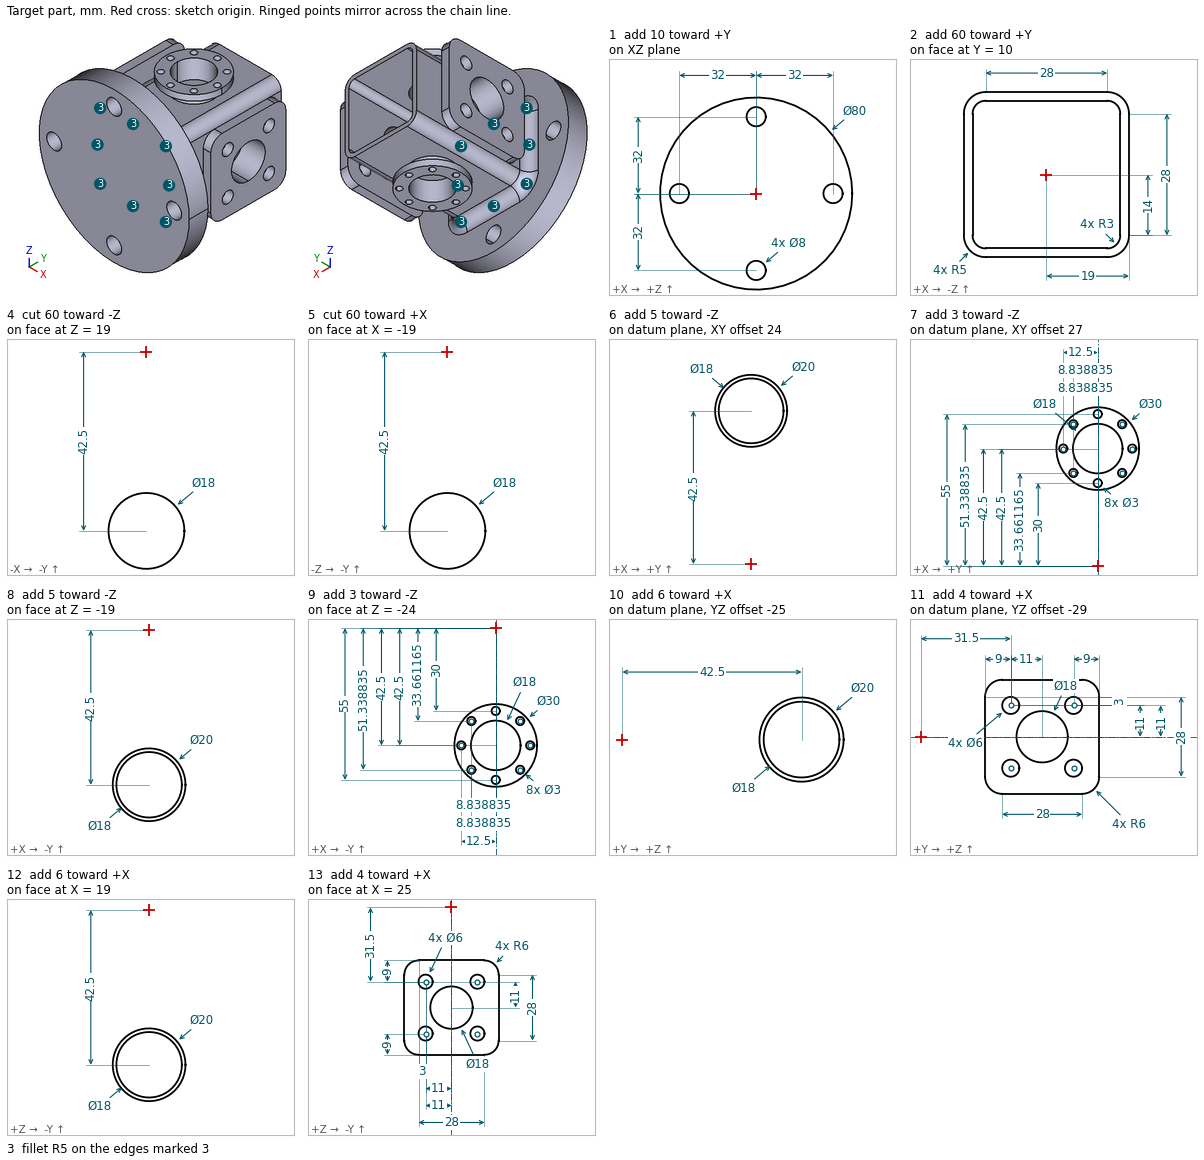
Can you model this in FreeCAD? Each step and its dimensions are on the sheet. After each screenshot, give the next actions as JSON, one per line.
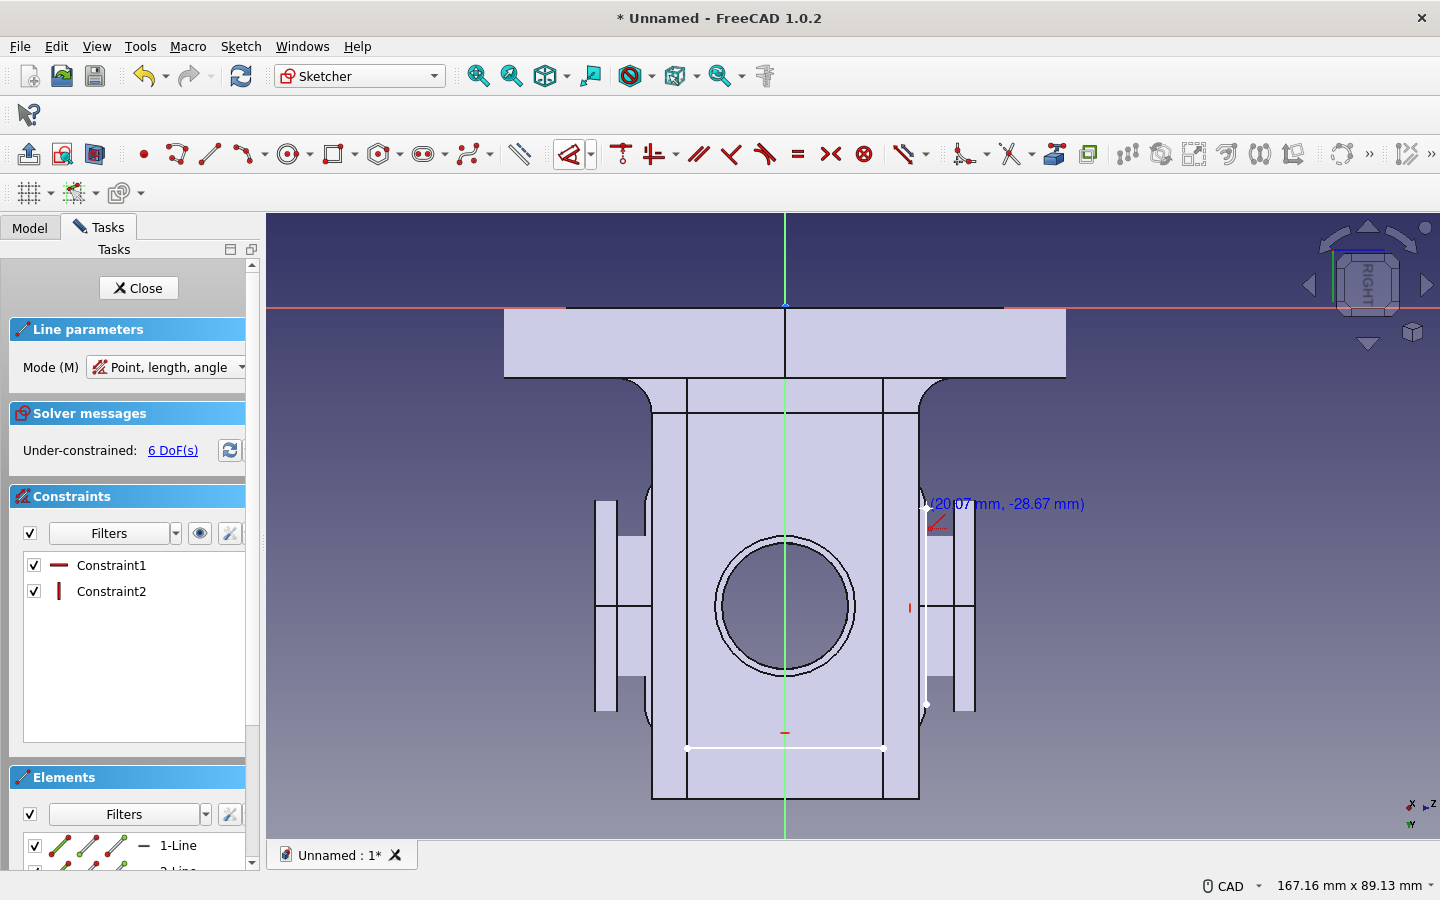
{"action": "left_click", "coordinate": [883, 466]}
{"action": "left_click", "coordinate": [687, 466]}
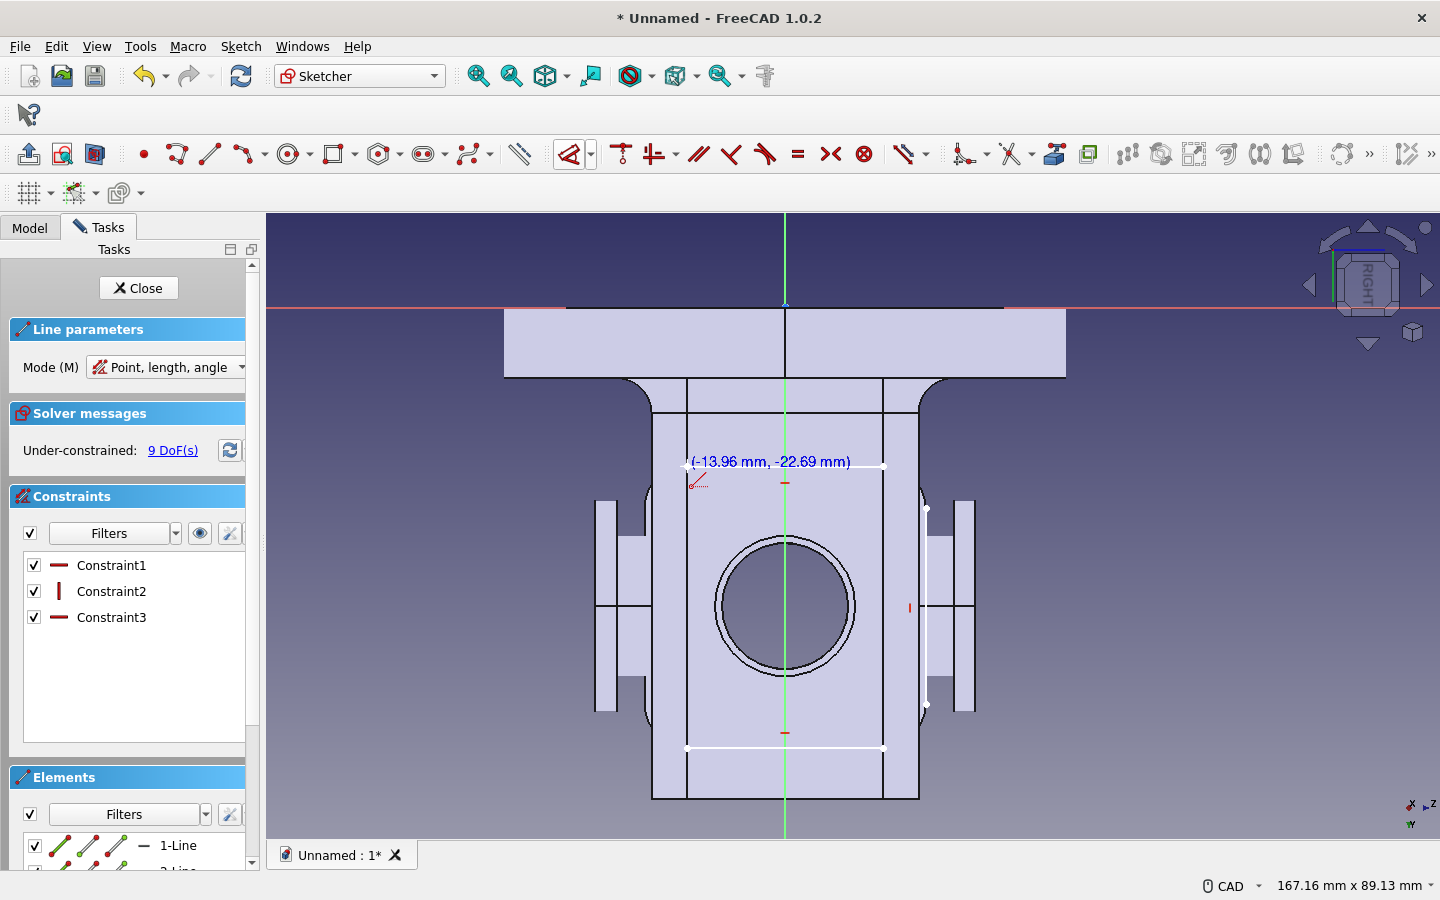
{"action": "left_click", "coordinate": [645, 508]}
{"action": "left_click", "coordinate": [645, 704]}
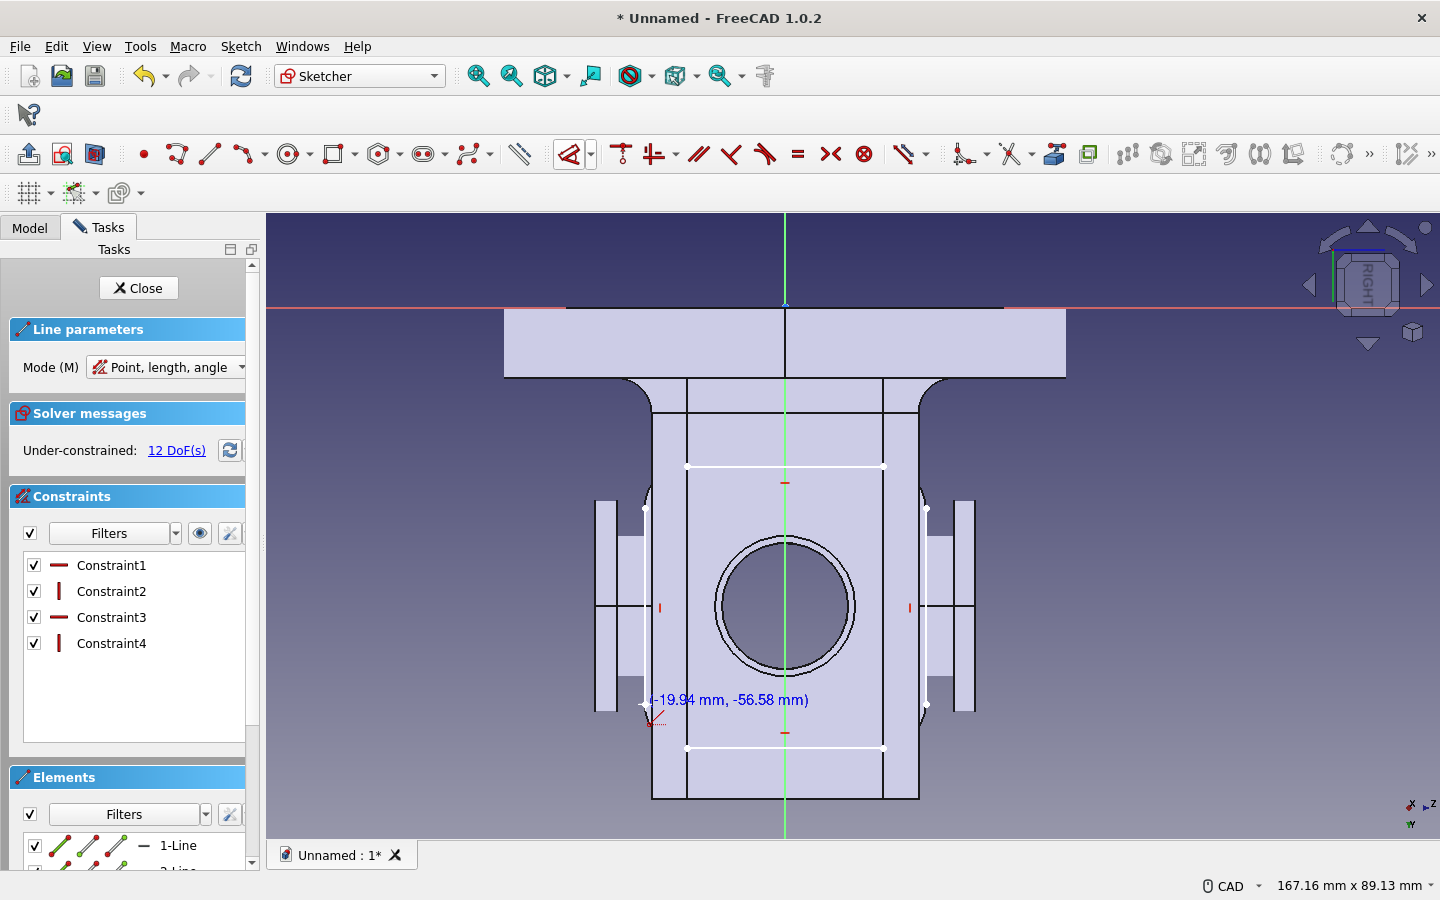
{"action": "left_click", "coordinate": [242, 154]}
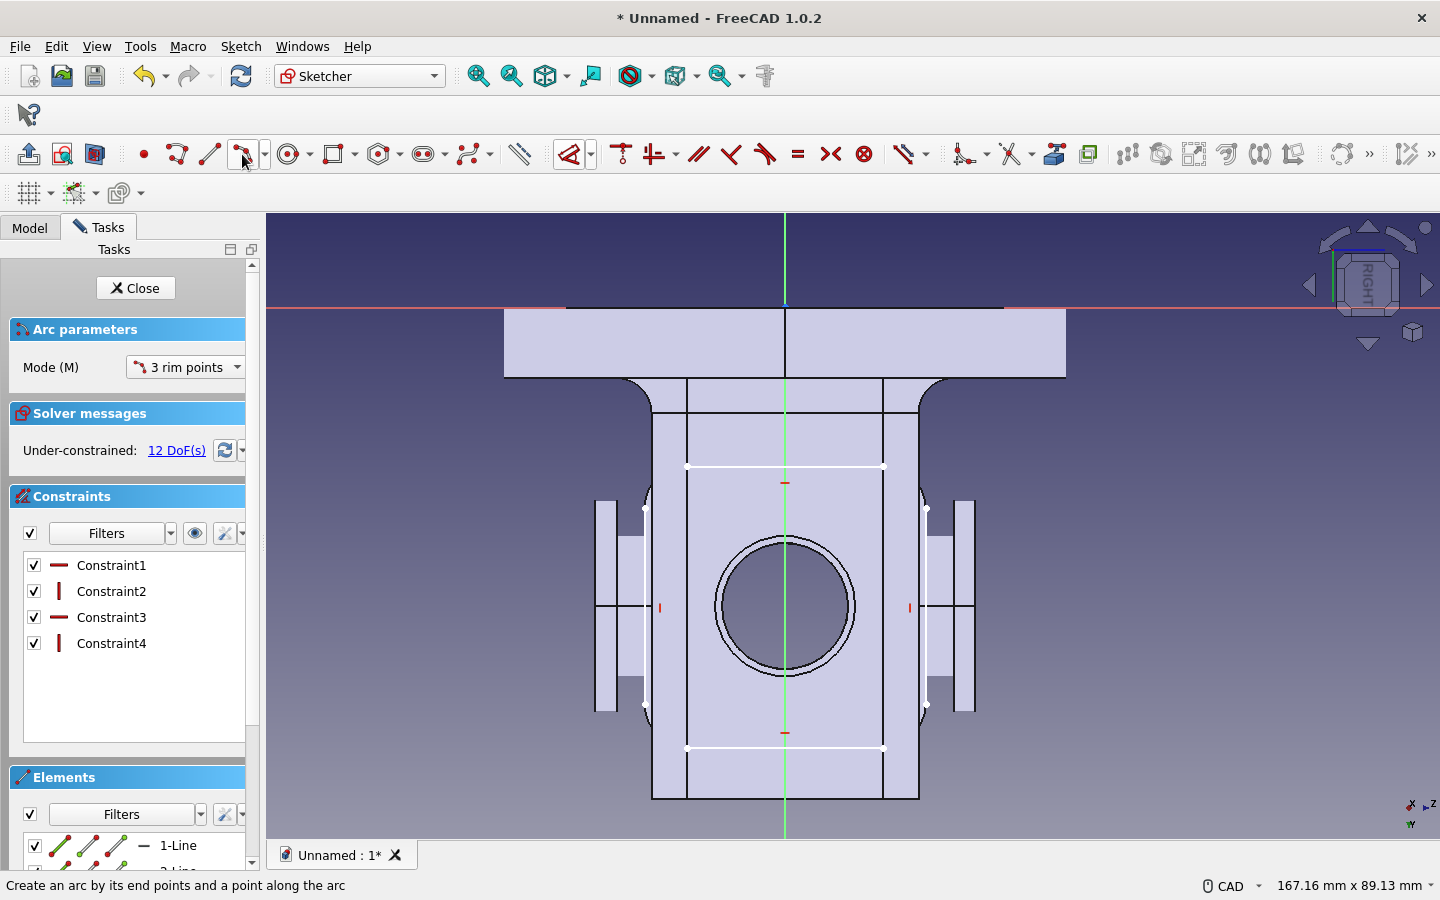
{"action": "left_click", "coordinate": [883, 748]}
{"action": "left_click", "coordinate": [926, 705]}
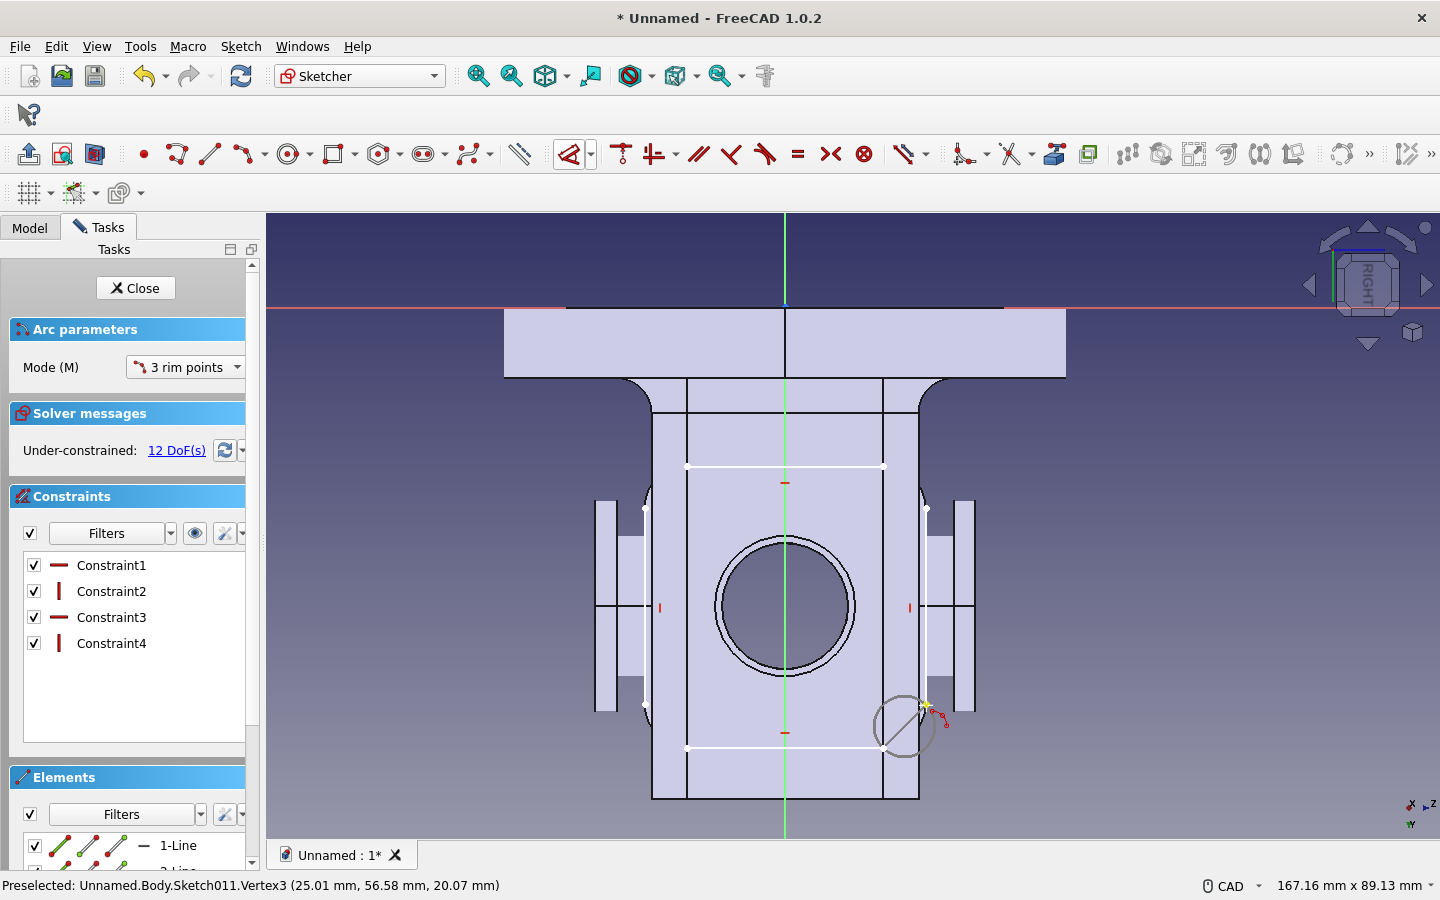
{"action": "scroll", "coordinate": [913, 734], "scroll_direction": "up", "scroll_amount": 2}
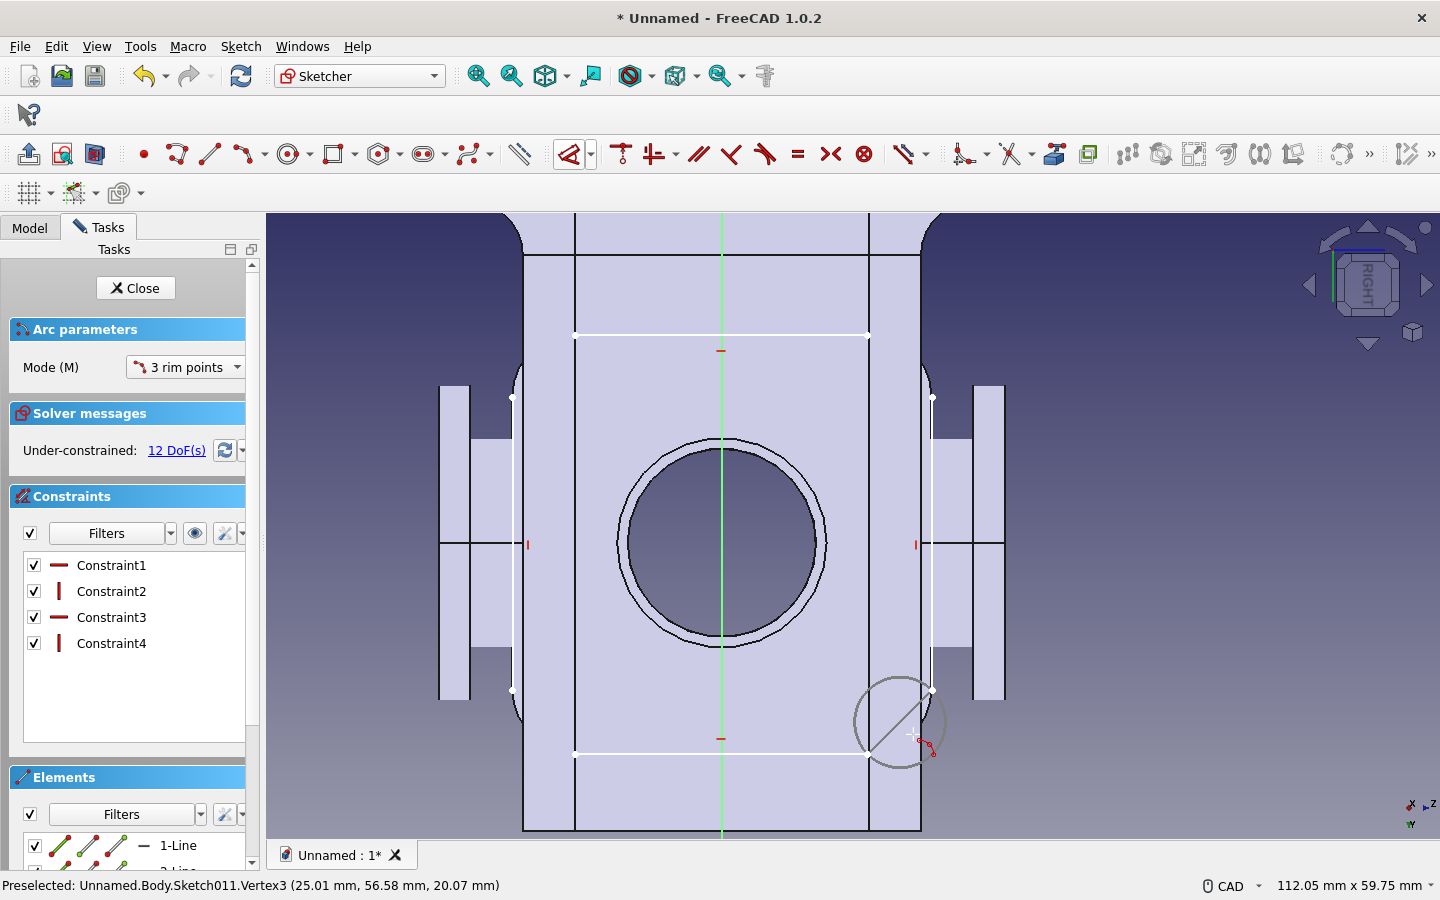
{"action": "left_click", "coordinate": [913, 734]}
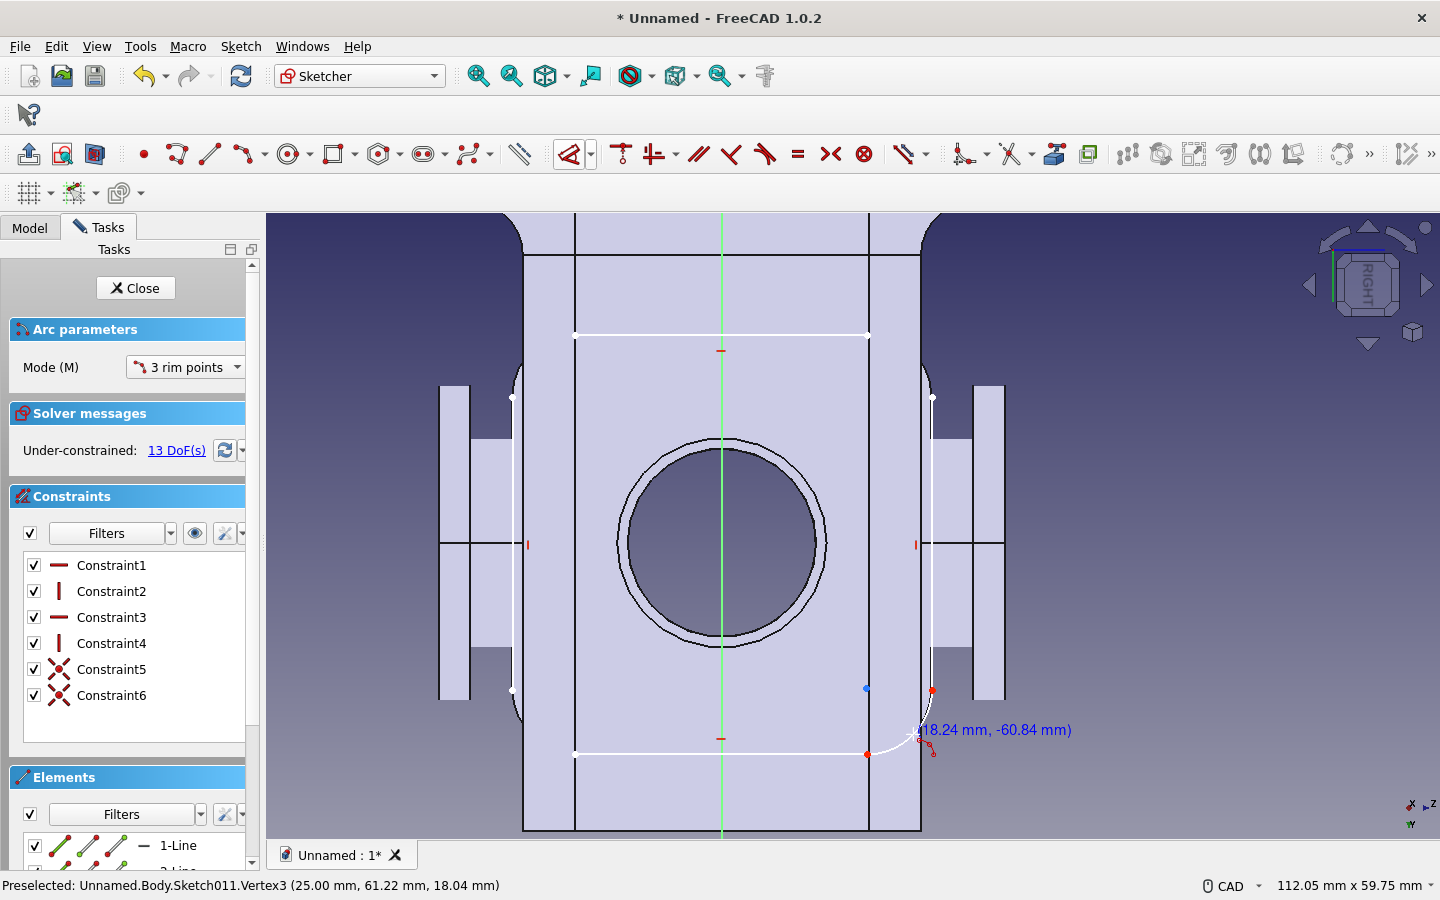
{"action": "left_click", "coordinate": [932, 398]}
{"action": "left_click", "coordinate": [868, 335]}
{"action": "left_click", "coordinate": [913, 352]}